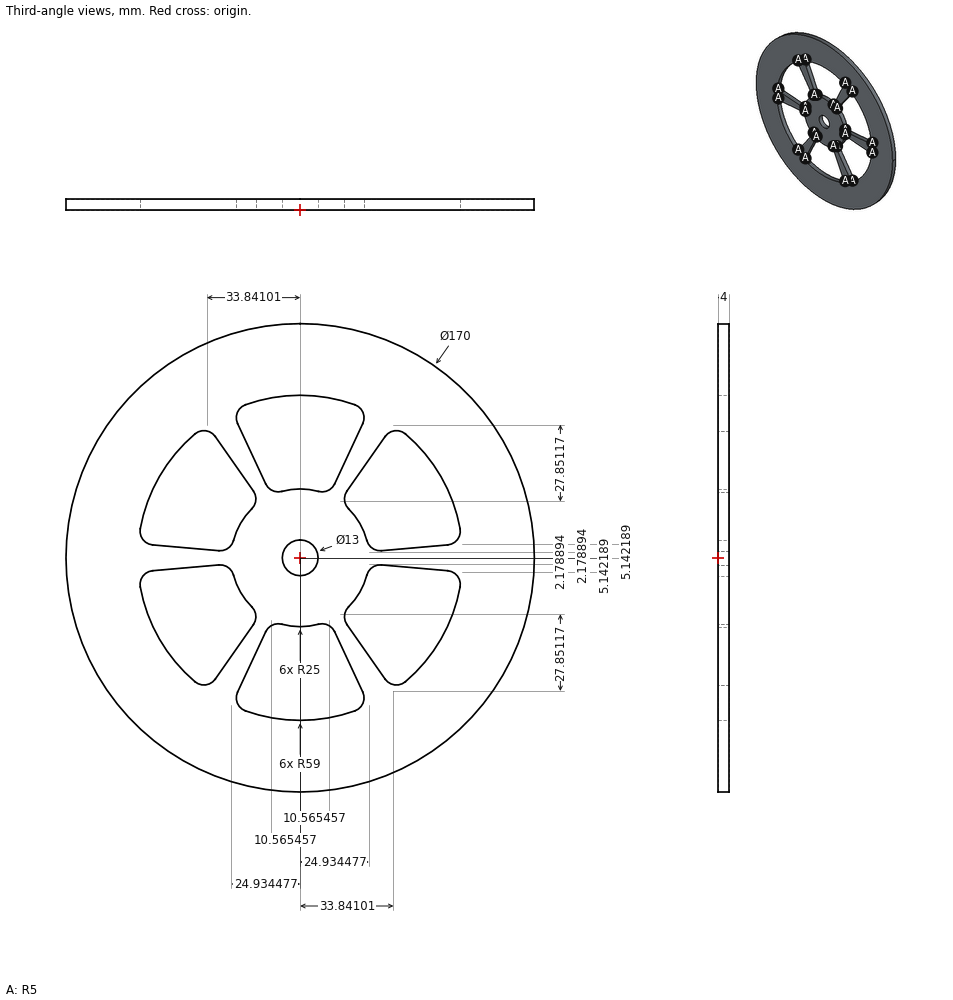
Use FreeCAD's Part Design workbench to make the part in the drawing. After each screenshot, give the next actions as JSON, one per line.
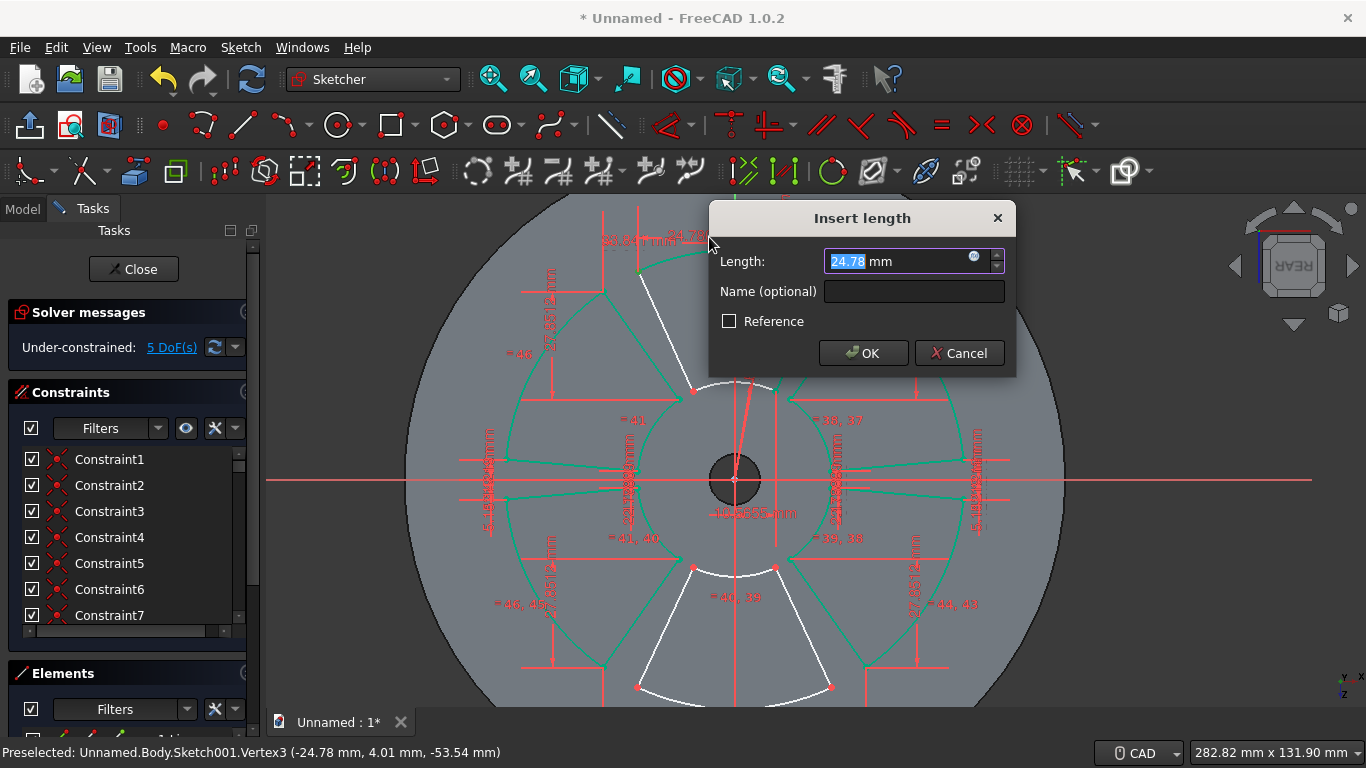
{"action": "type", "text": "24.934477"}
{"action": "key", "text": "Return"}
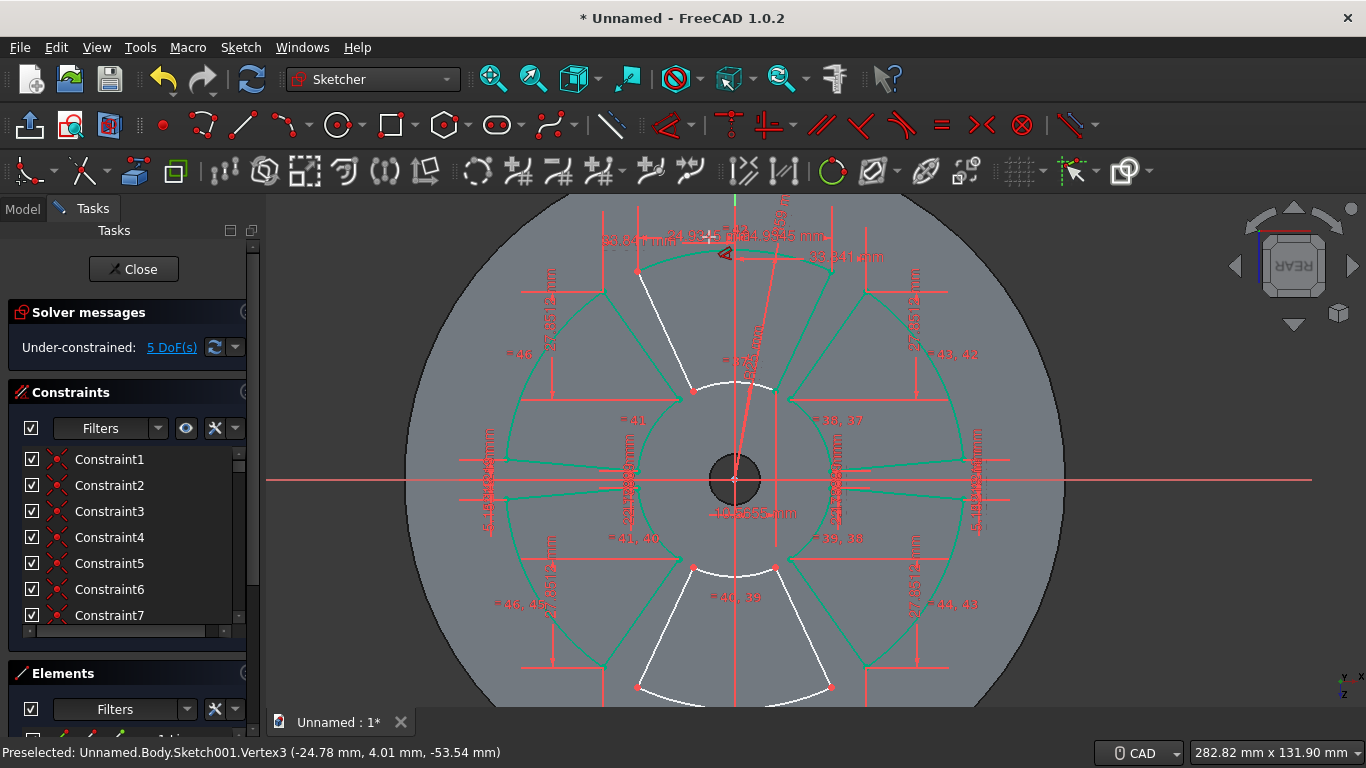
{"action": "left_click", "coordinate": [693, 392]}
{"action": "left_click", "coordinate": [714, 538]}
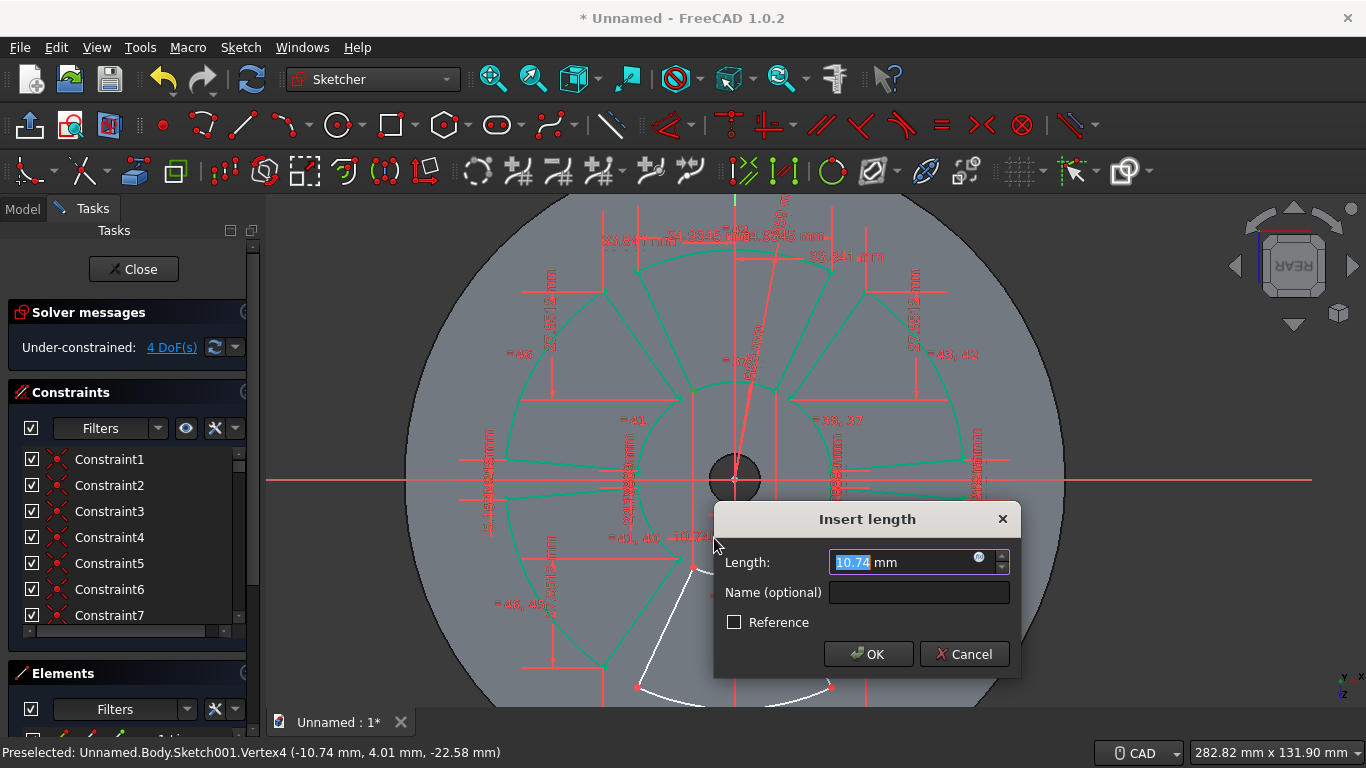
{"action": "type", "text": "10.565457"}
{"action": "key", "text": "Return"}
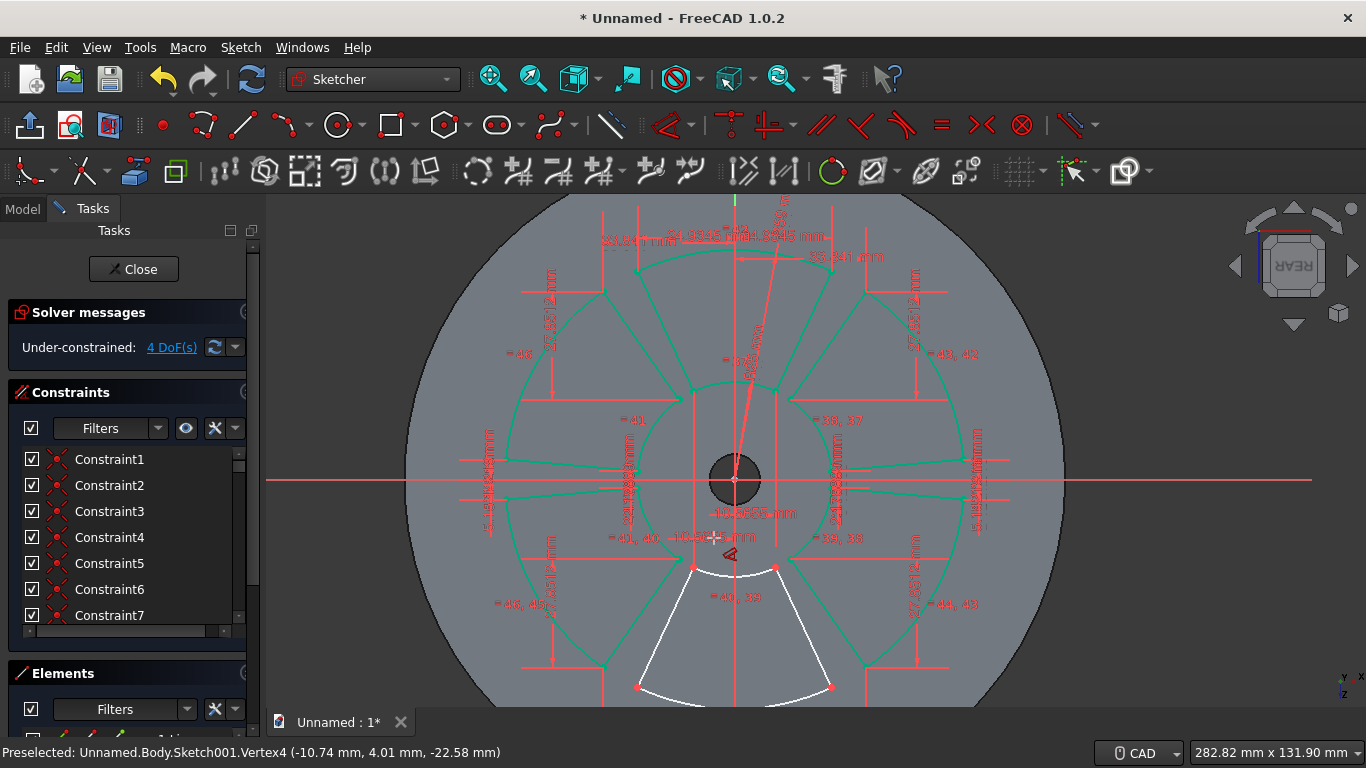
{"action": "scroll", "coordinate": [773, 391], "scroll_direction": "down", "scroll_amount": 2}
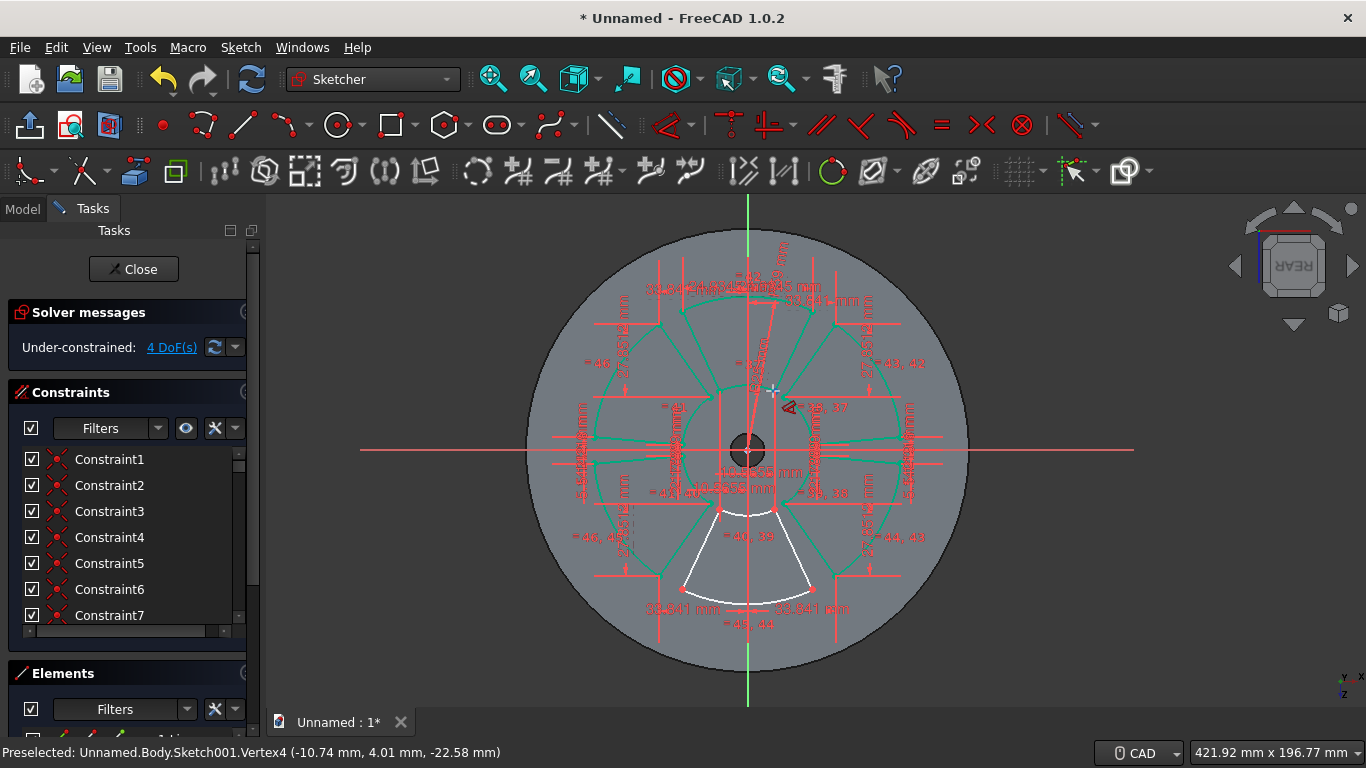
{"action": "left_click", "coordinate": [812, 590]}
{"action": "left_click", "coordinate": [780, 416]}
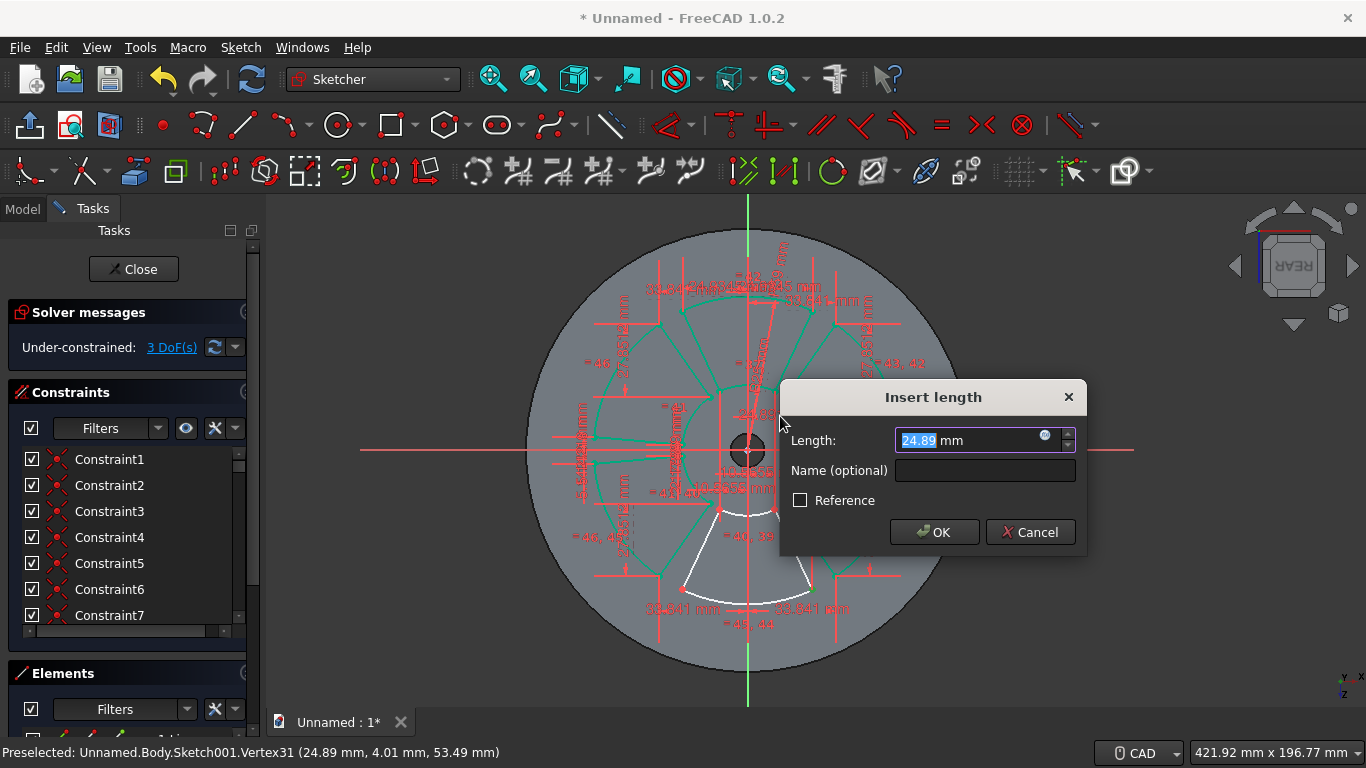
{"action": "type", "text": "24.934477"}
{"action": "key", "text": "Return"}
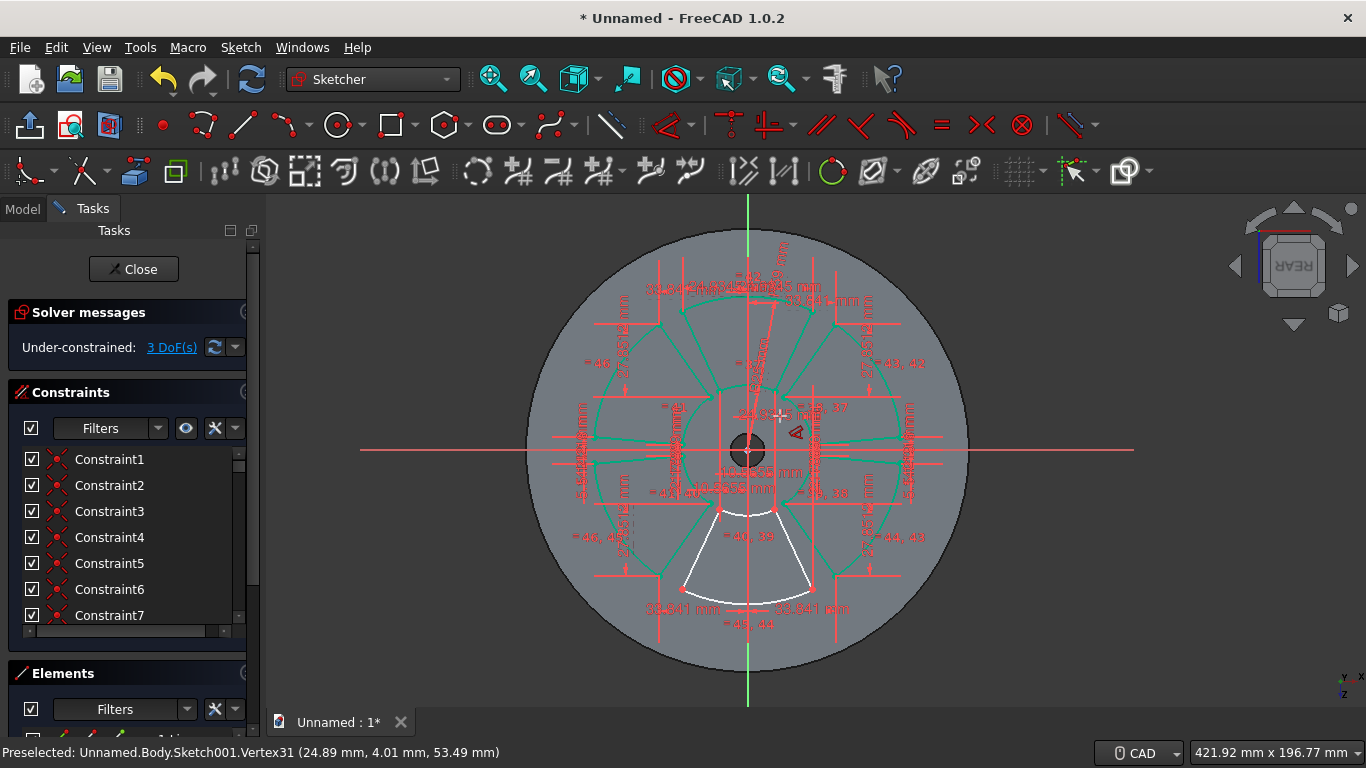
{"action": "scroll", "coordinate": [775, 510], "scroll_direction": "up", "scroll_amount": 2}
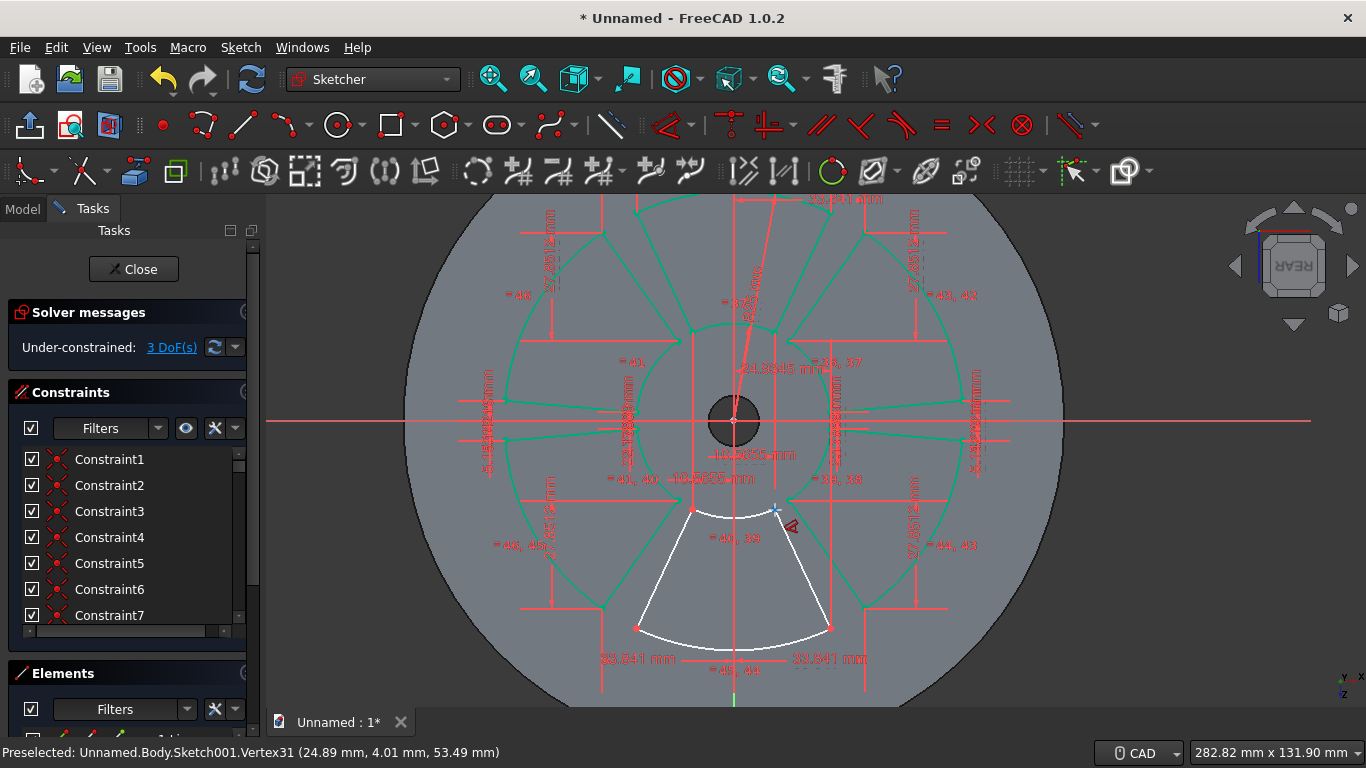
{"action": "left_click", "coordinate": [775, 509]}
{"action": "left_click", "coordinate": [754, 543]}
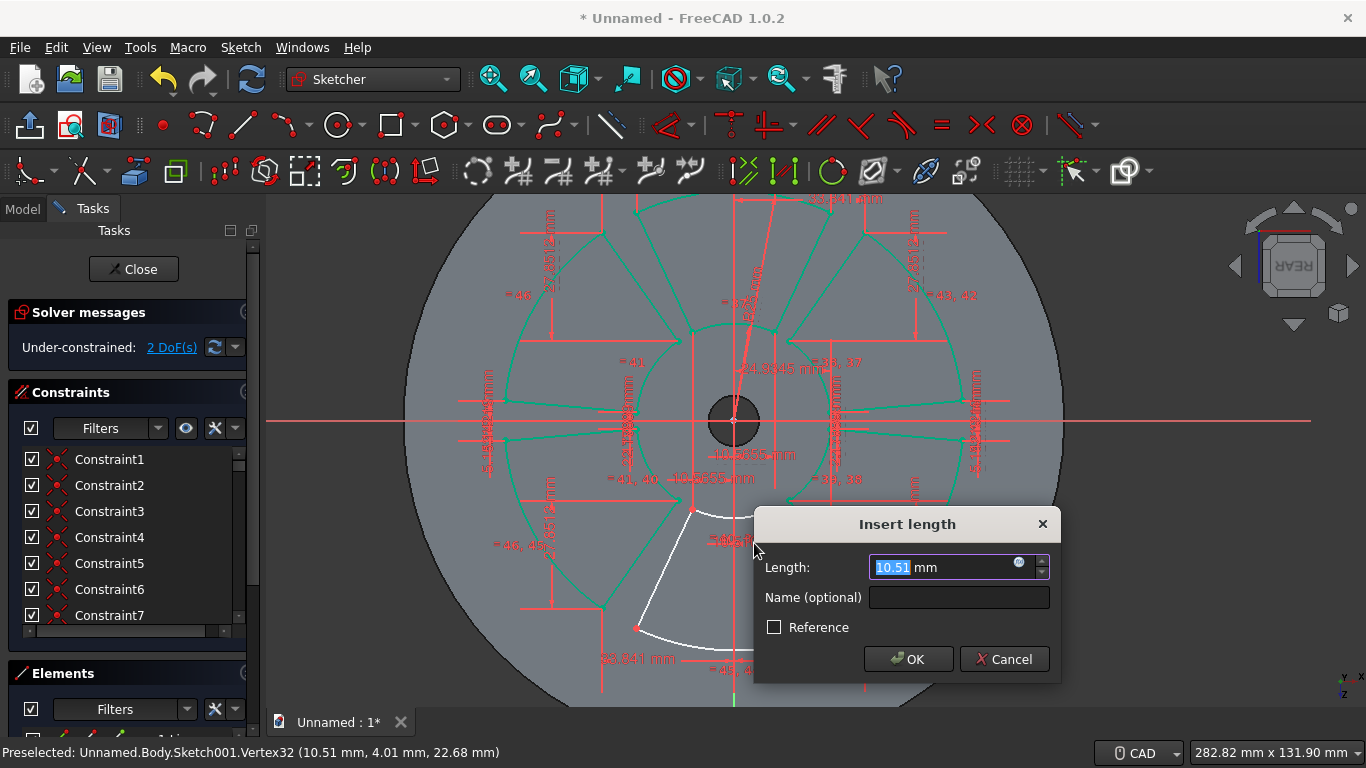
{"action": "type", "text": "10.565457"}
{"action": "key", "text": "Return"}